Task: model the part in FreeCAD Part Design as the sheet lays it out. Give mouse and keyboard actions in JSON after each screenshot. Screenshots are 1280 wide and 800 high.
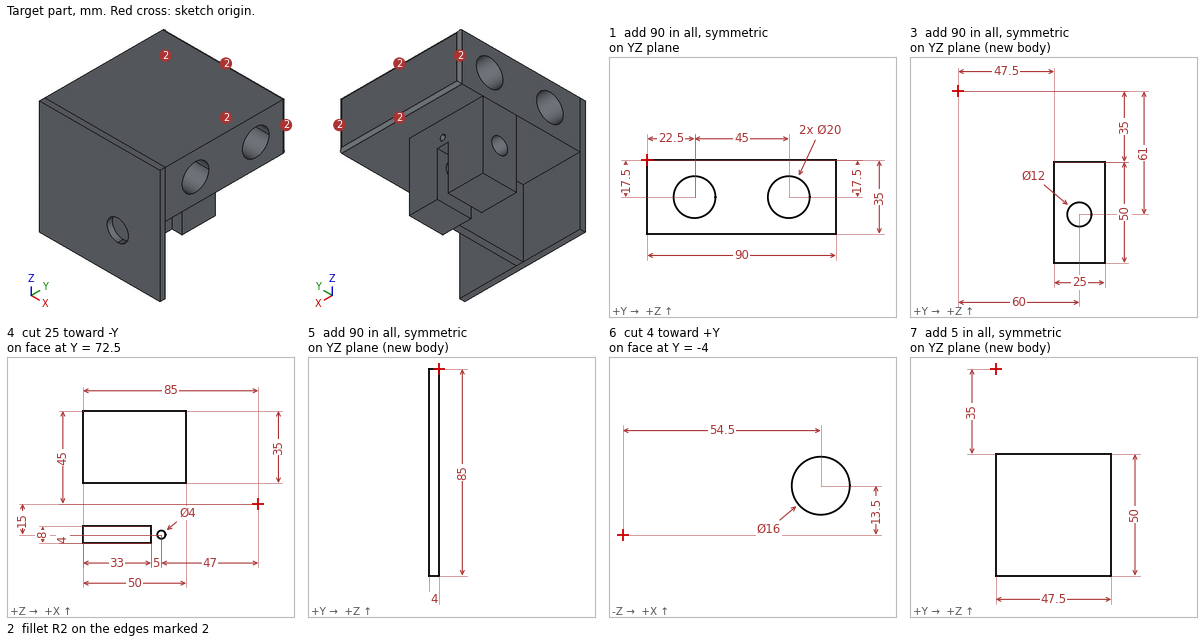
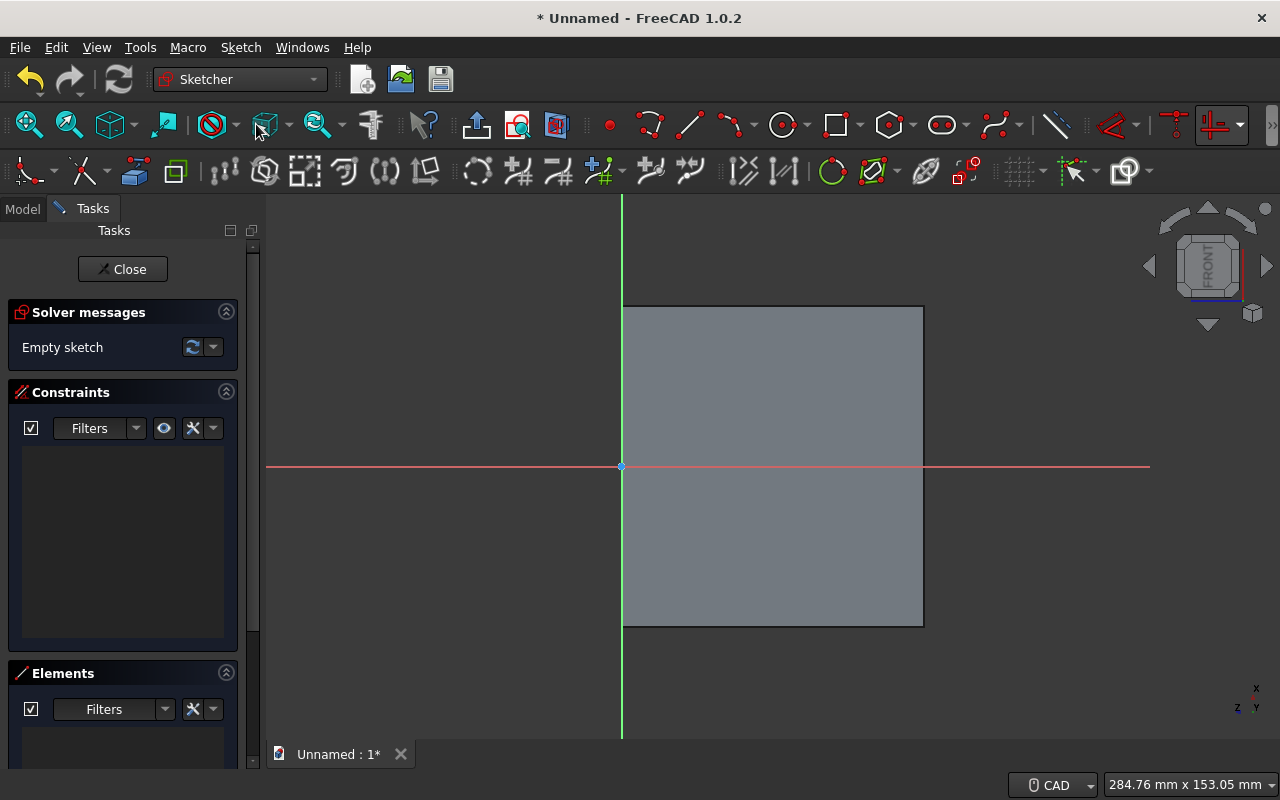
{"action": "scroll", "coordinate": [838, 409], "scroll_direction": "up", "scroll_amount": 9}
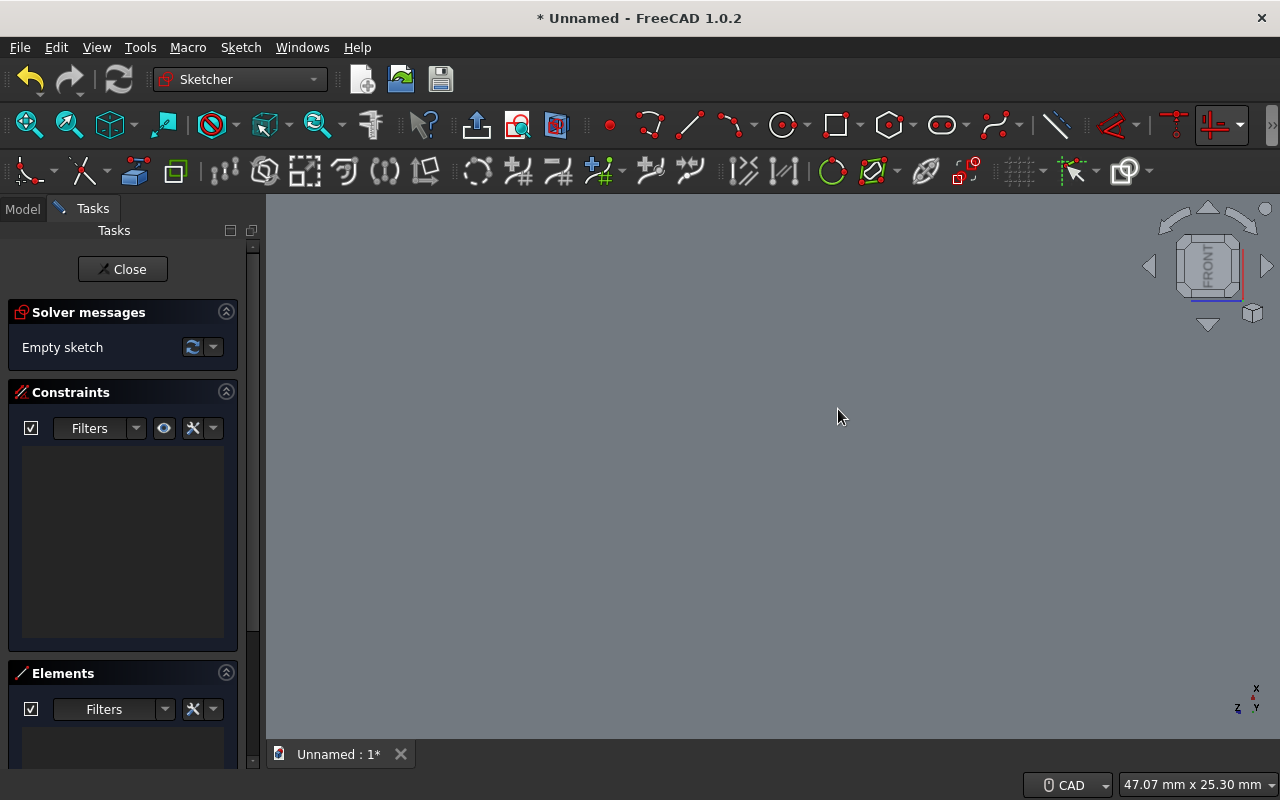
{"action": "left_click", "coordinate": [784, 126]}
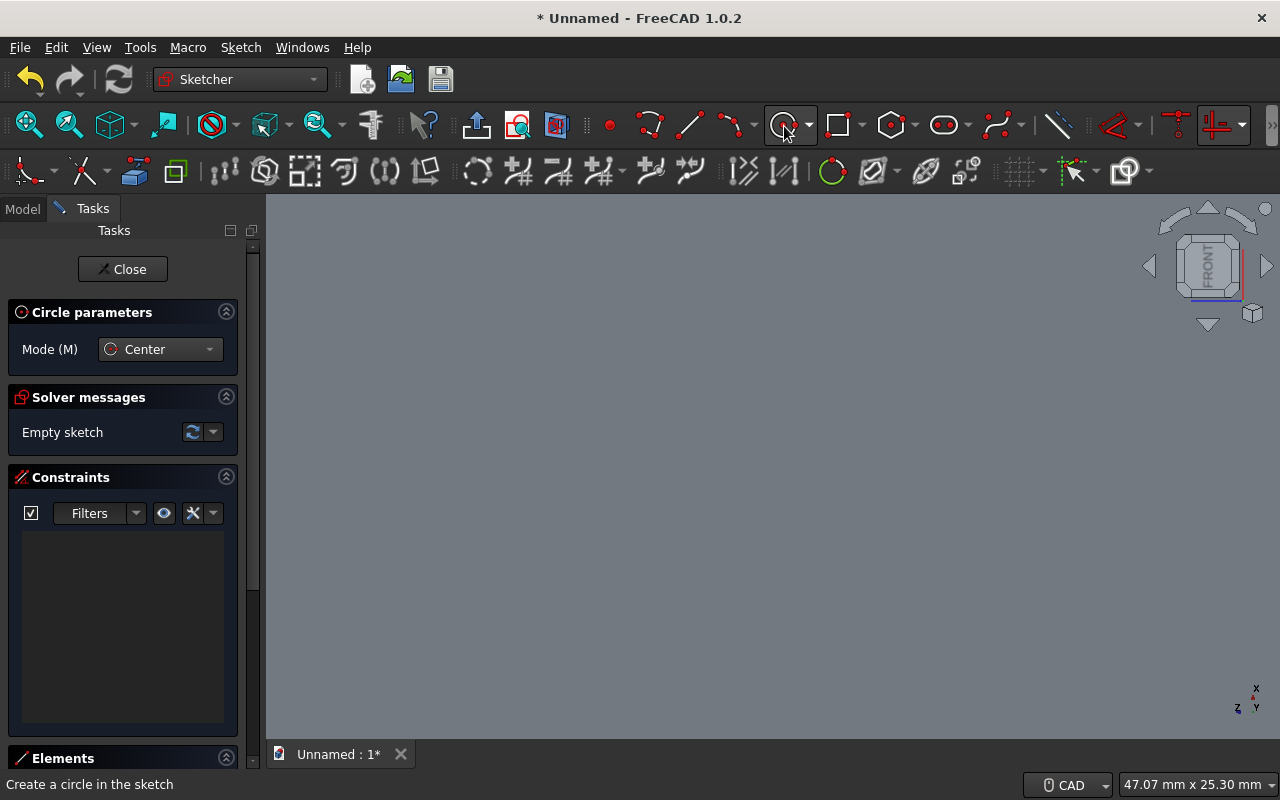
{"action": "left_click", "coordinate": [700, 464]}
{"action": "mouse_move", "coordinate": [822, 342]}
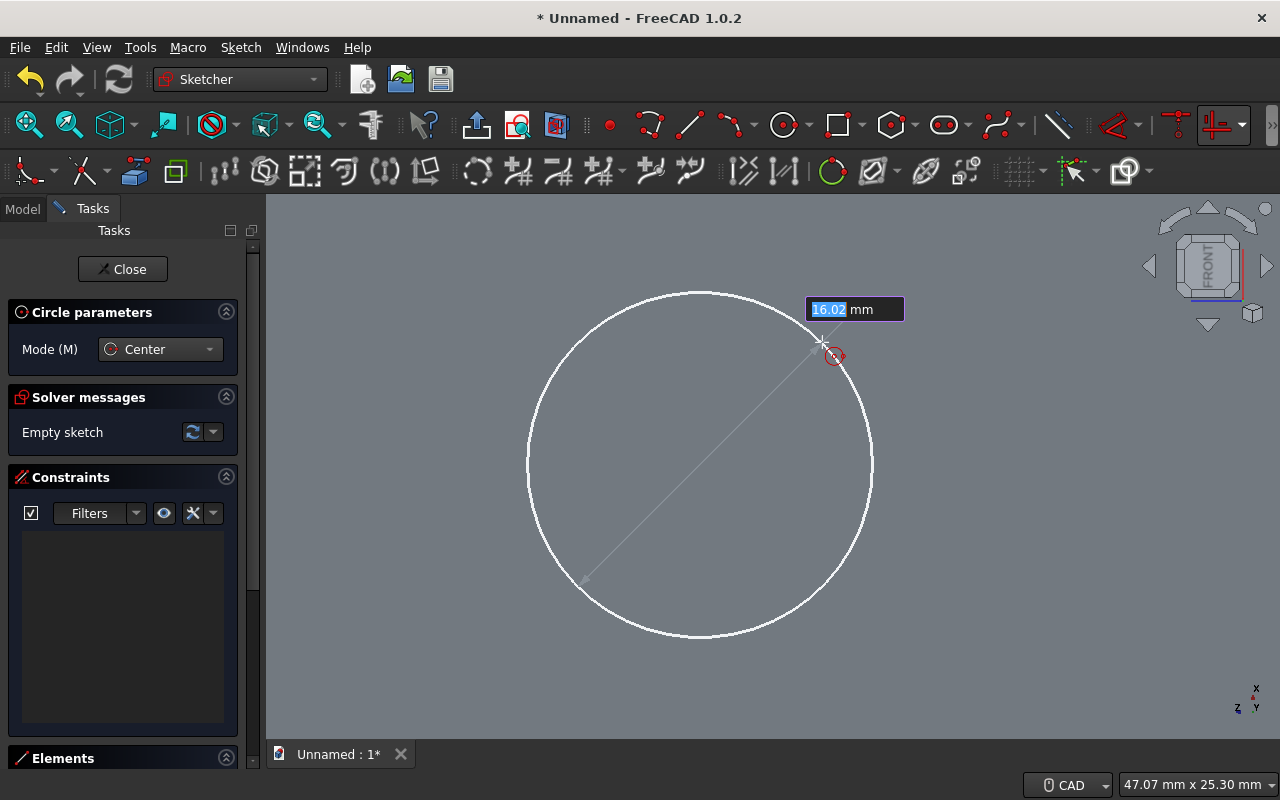
{"action": "type", "text": "16"}
{"action": "key", "text": "Return"}
{"action": "key", "text": "Escape"}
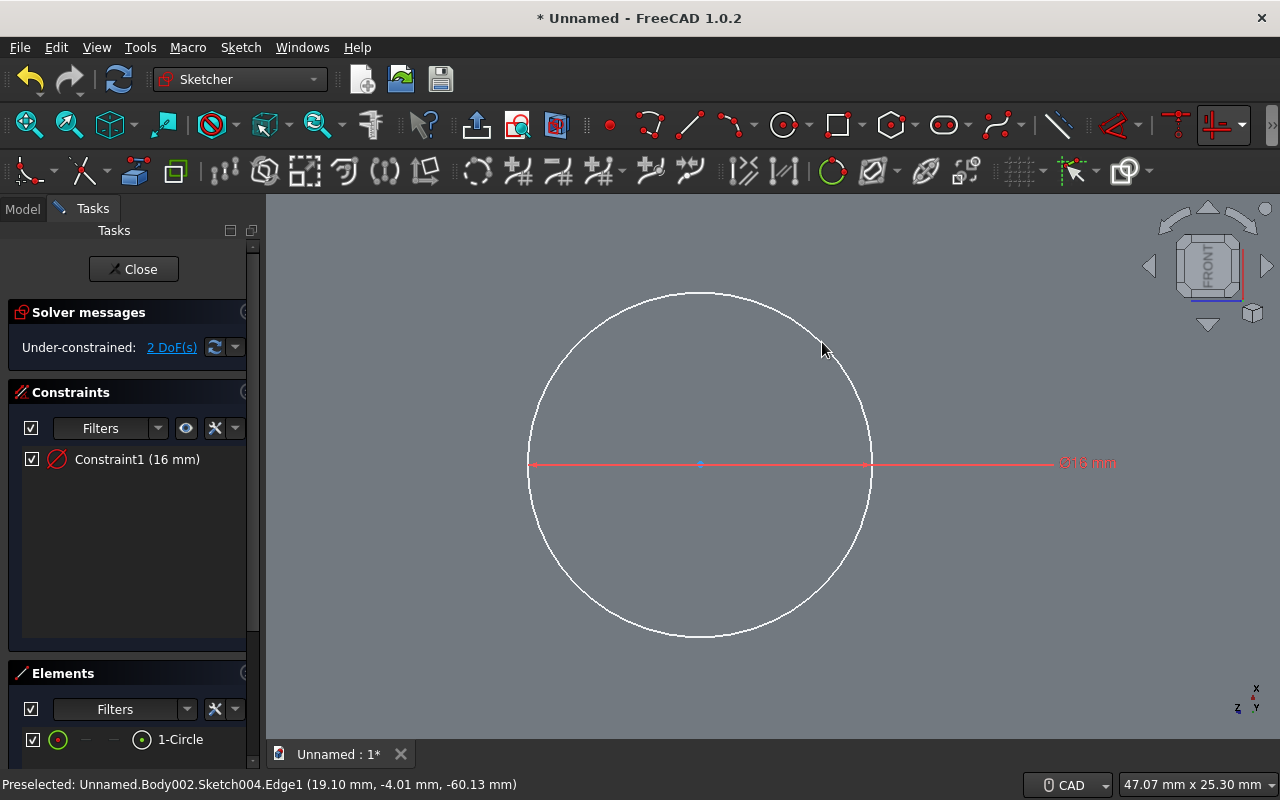
{"action": "left_click", "coordinate": [1114, 126]}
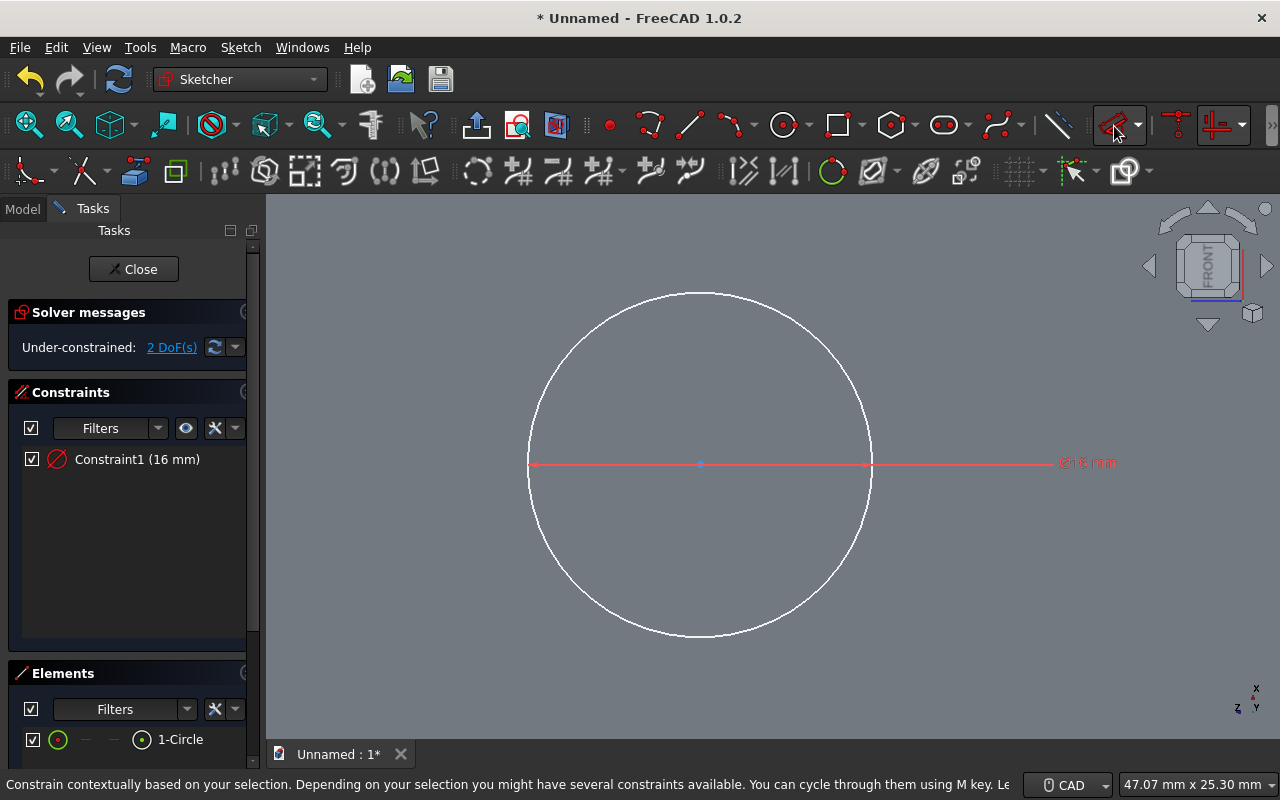
{"action": "left_click", "coordinate": [700, 465]}
{"action": "left_click", "coordinate": [497, 431]}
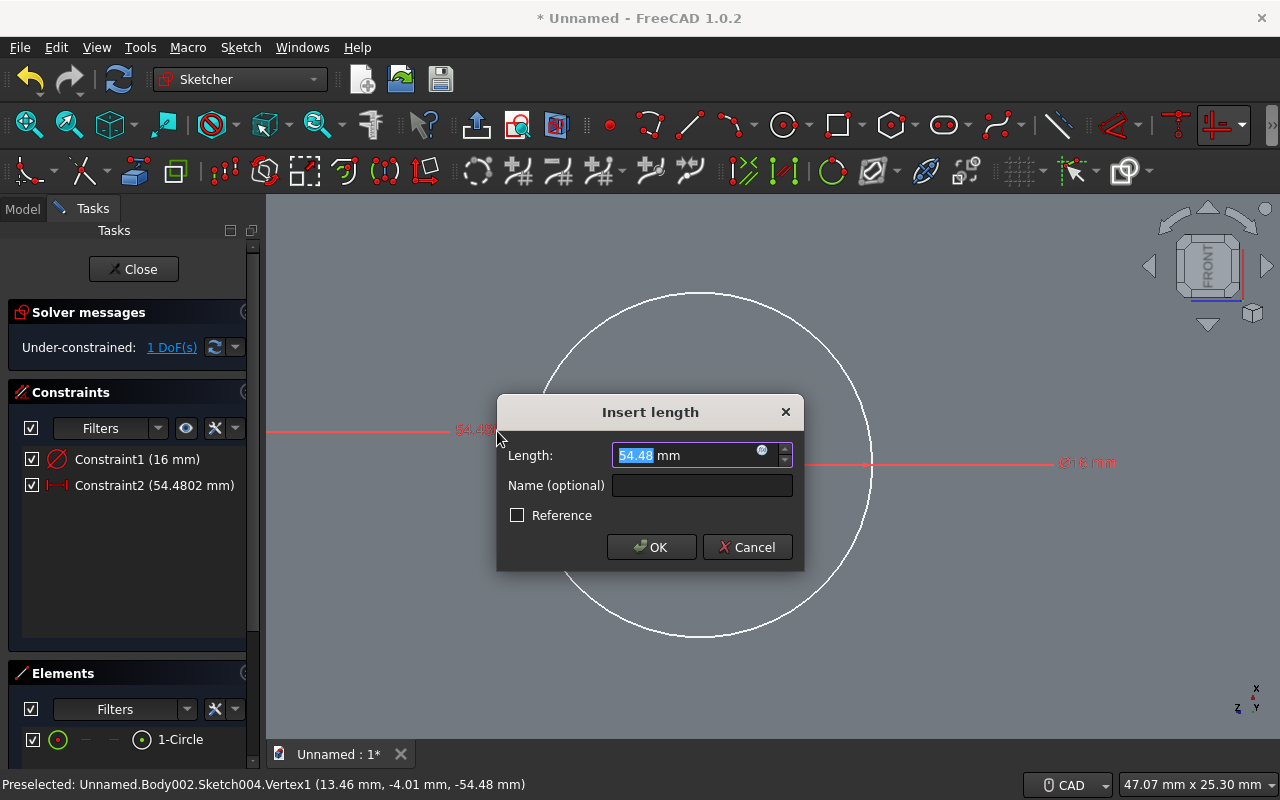
{"action": "type", "text": "54.5"}
{"action": "key", "text": "Return"}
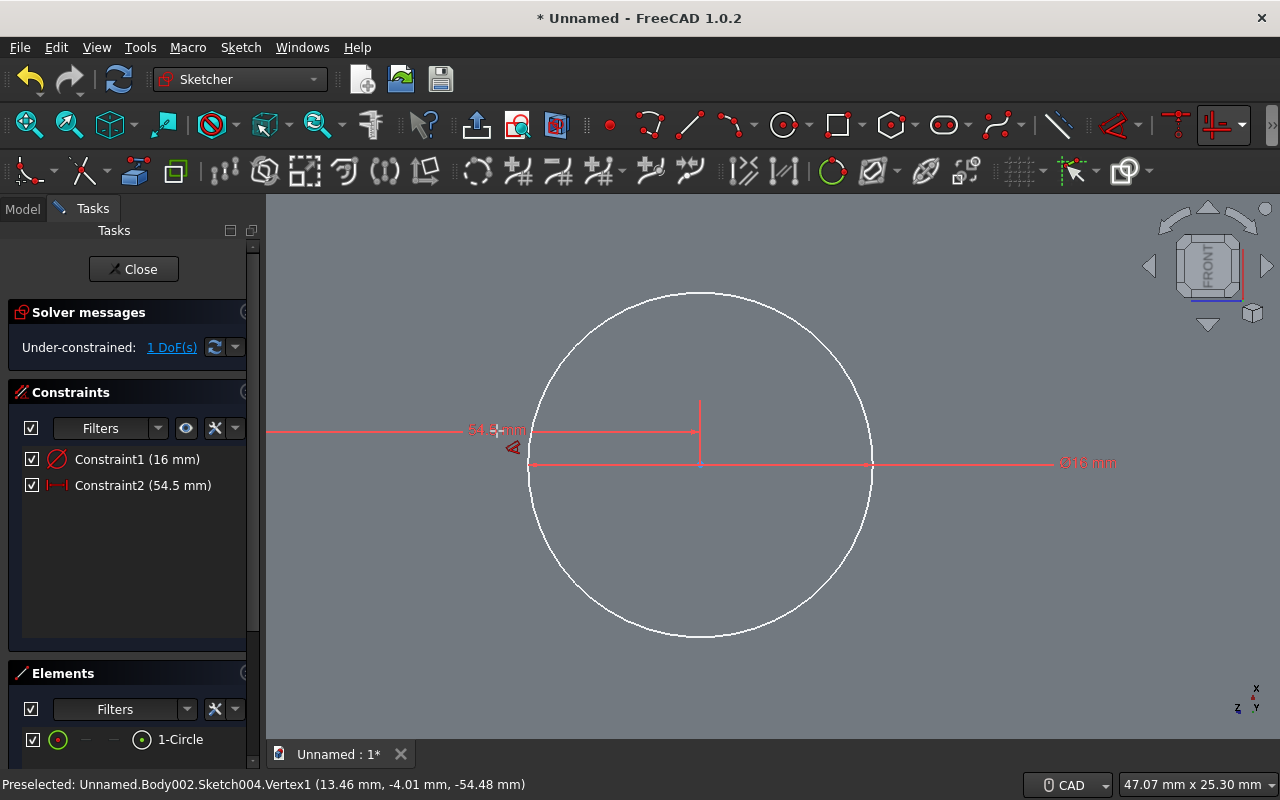
{"action": "left_click", "coordinate": [700, 465]}
{"action": "left_click", "coordinate": [734, 588]}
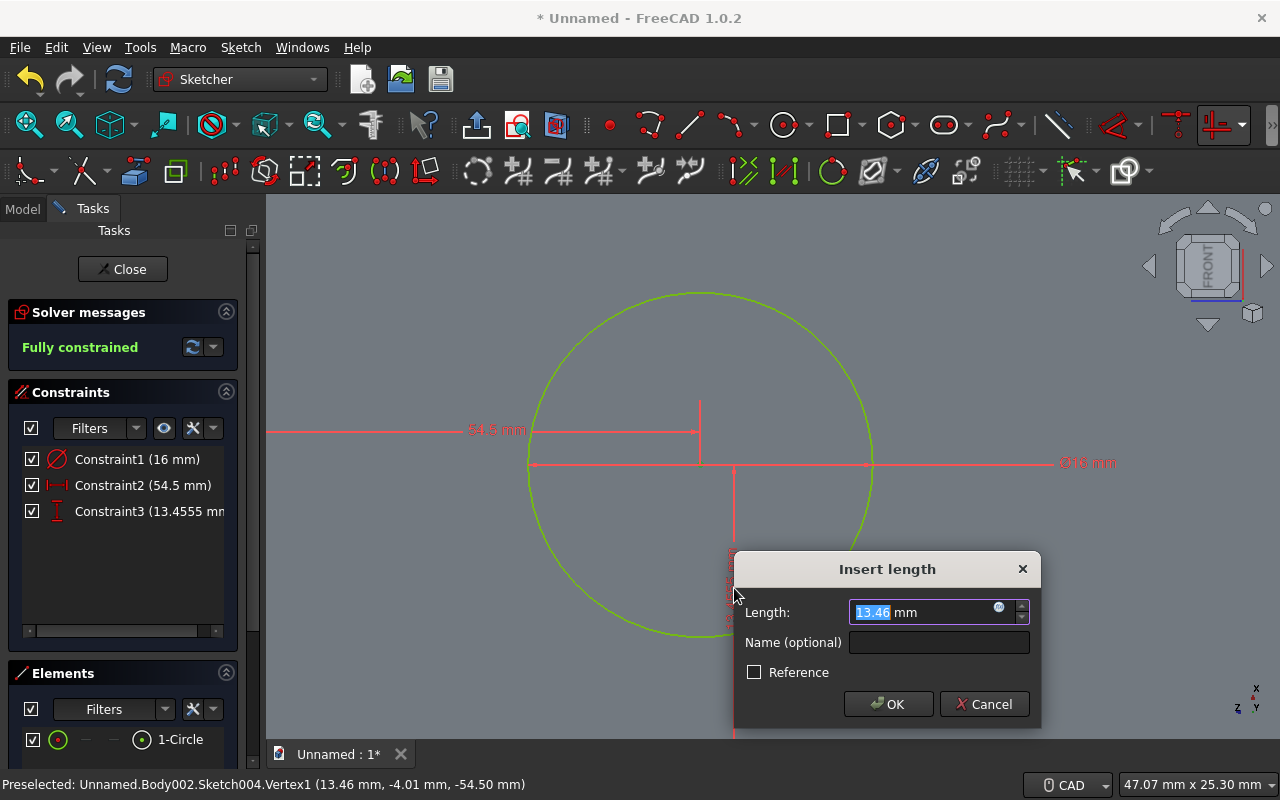
{"action": "type", "text": "13.5"}
{"action": "key", "text": "Return"}
{"action": "key", "text": "Escape"}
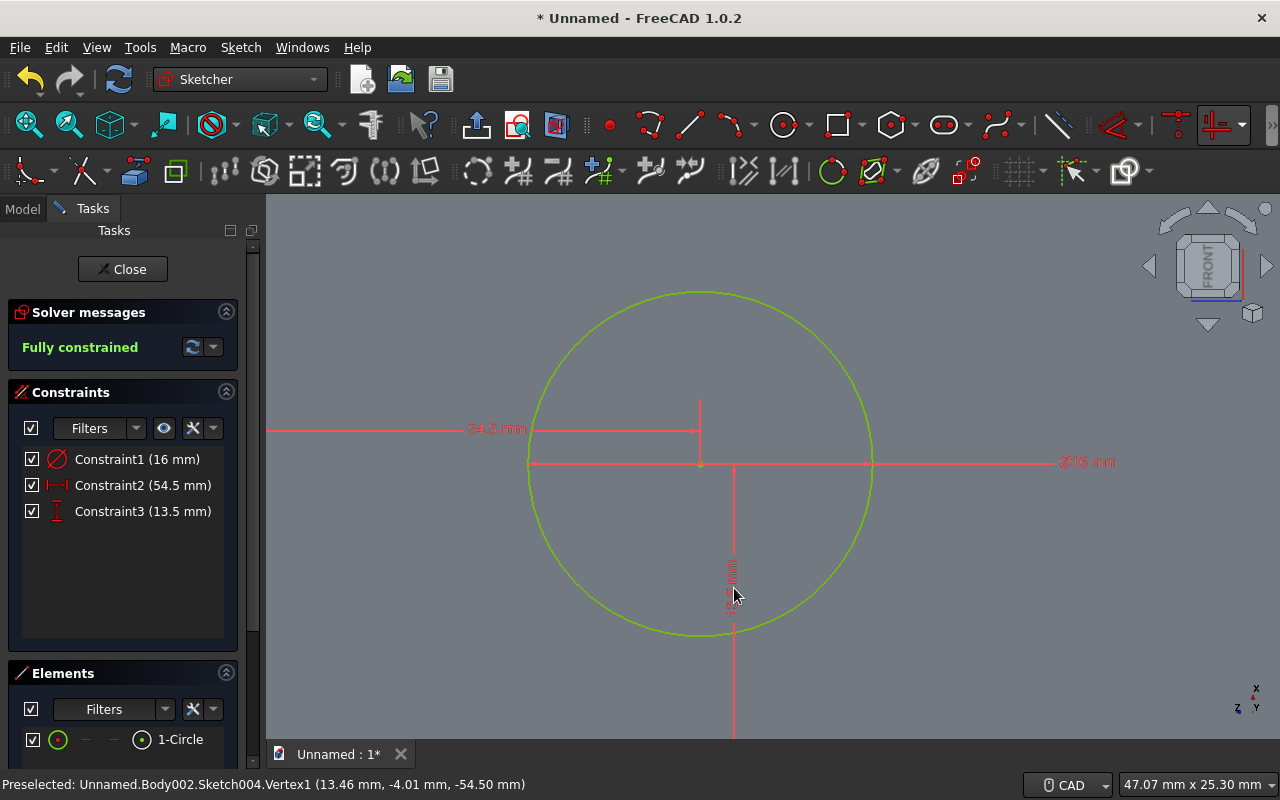
{"action": "left_click", "coordinate": [123, 269]}